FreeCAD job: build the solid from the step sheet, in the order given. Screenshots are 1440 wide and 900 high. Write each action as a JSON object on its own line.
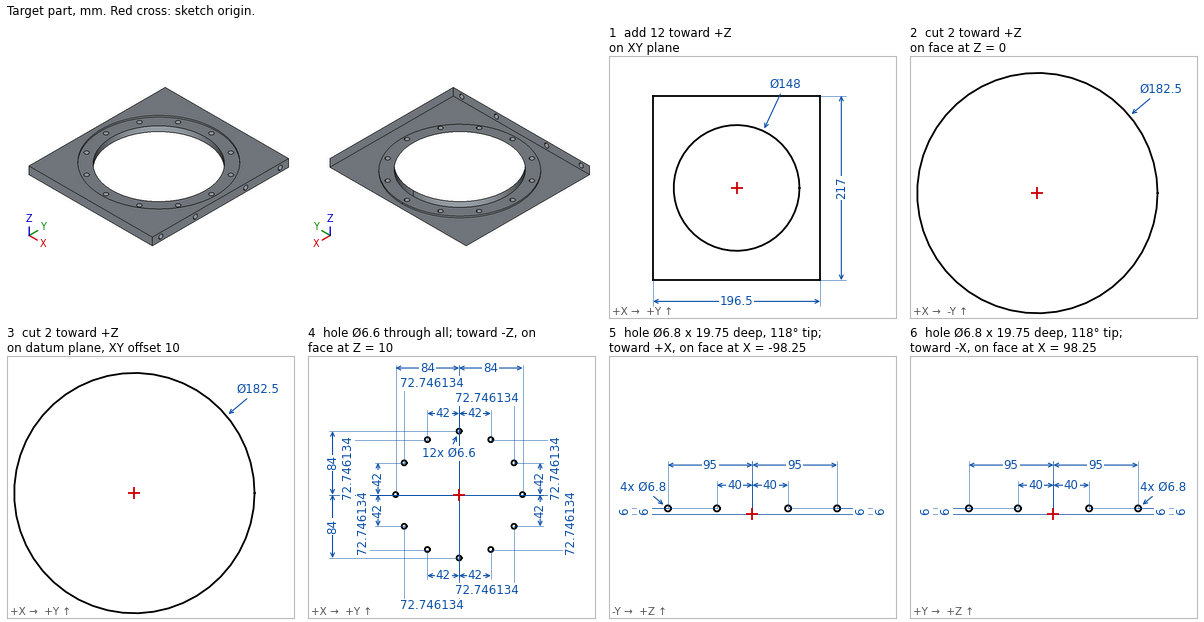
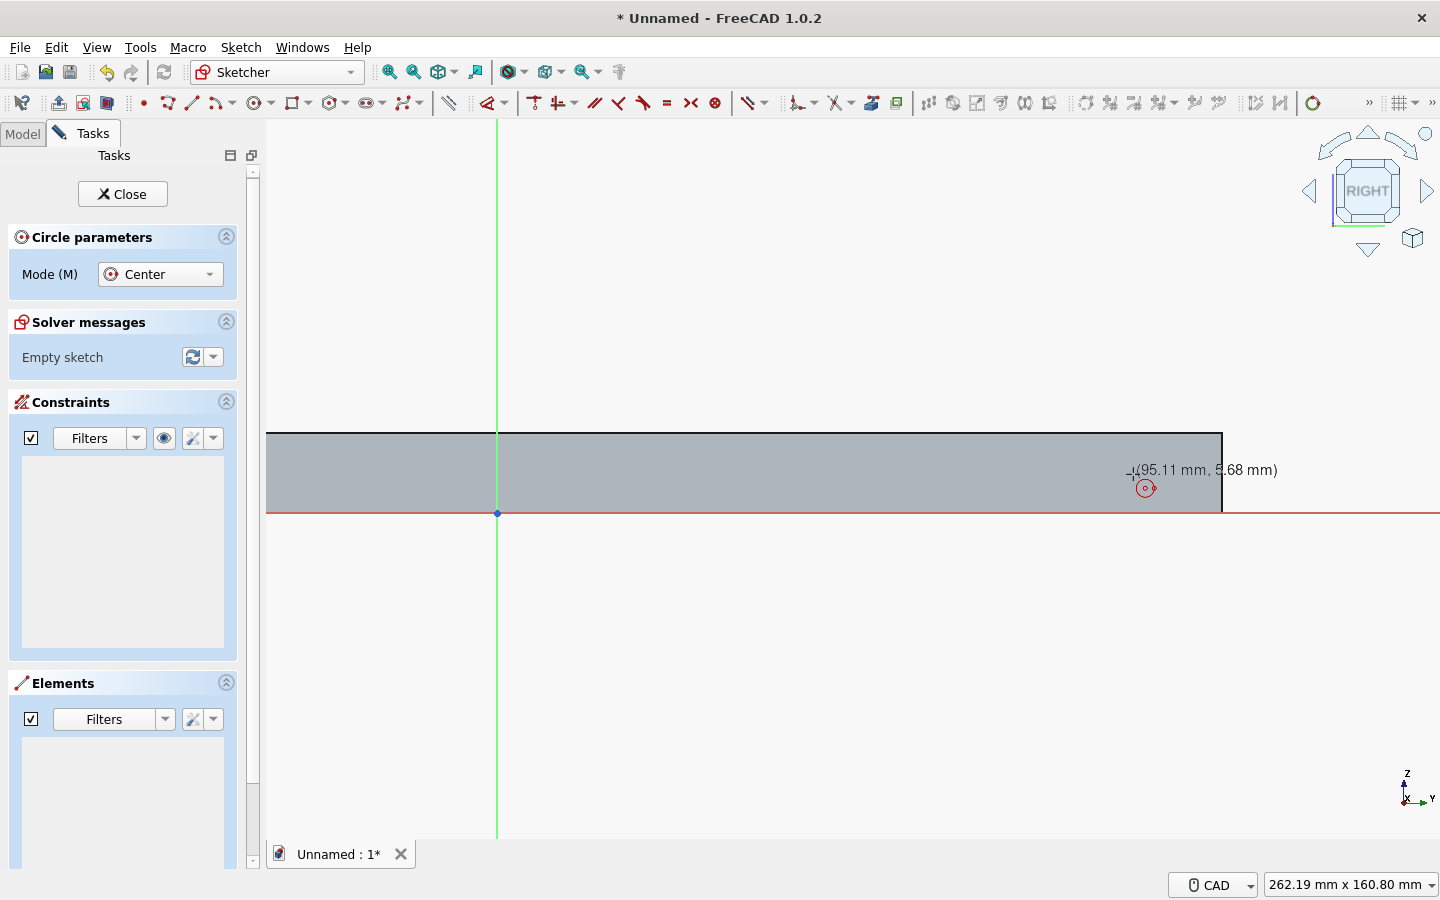
{"action": "left_click", "coordinate": [1132, 473]}
{"action": "mouse_move", "coordinate": [1148, 457]}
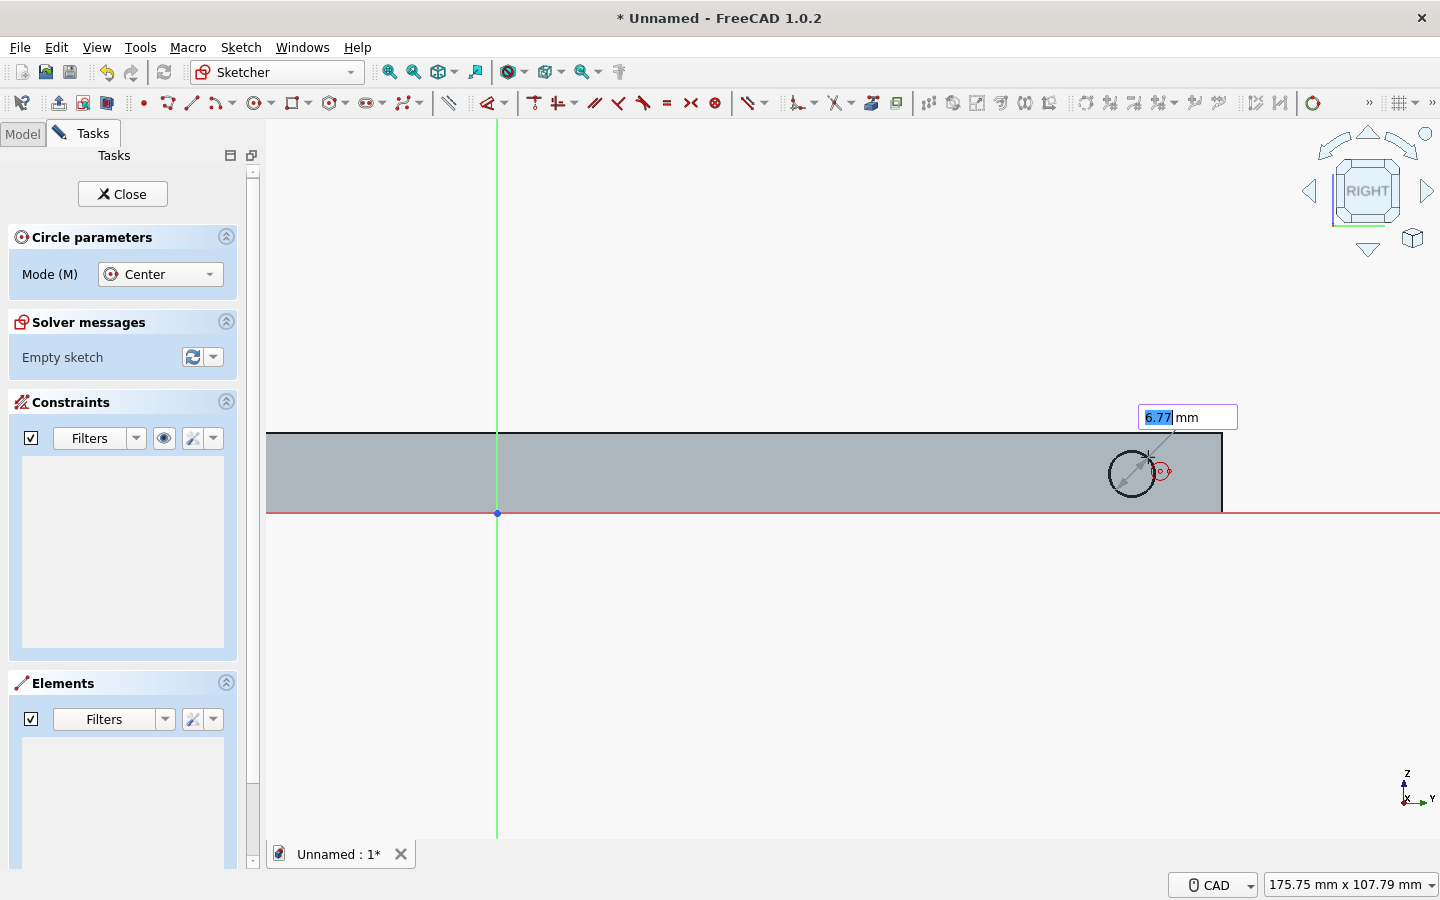
{"action": "type", "text": "6.8"}
{"action": "key", "text": "Return"}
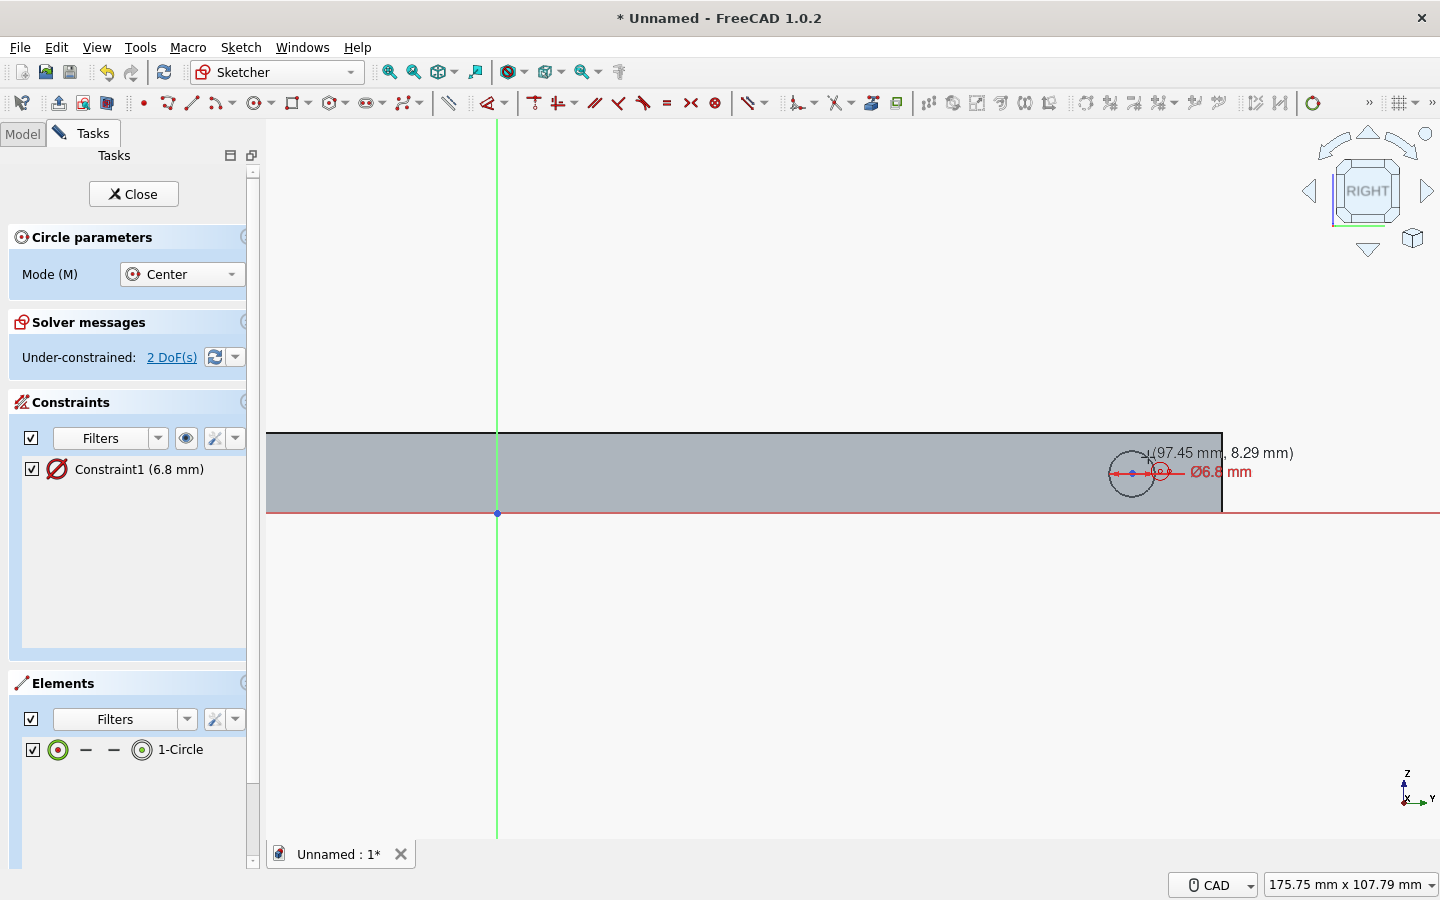
{"action": "left_click", "coordinate": [764, 473]}
{"action": "mouse_move", "coordinate": [780, 457]}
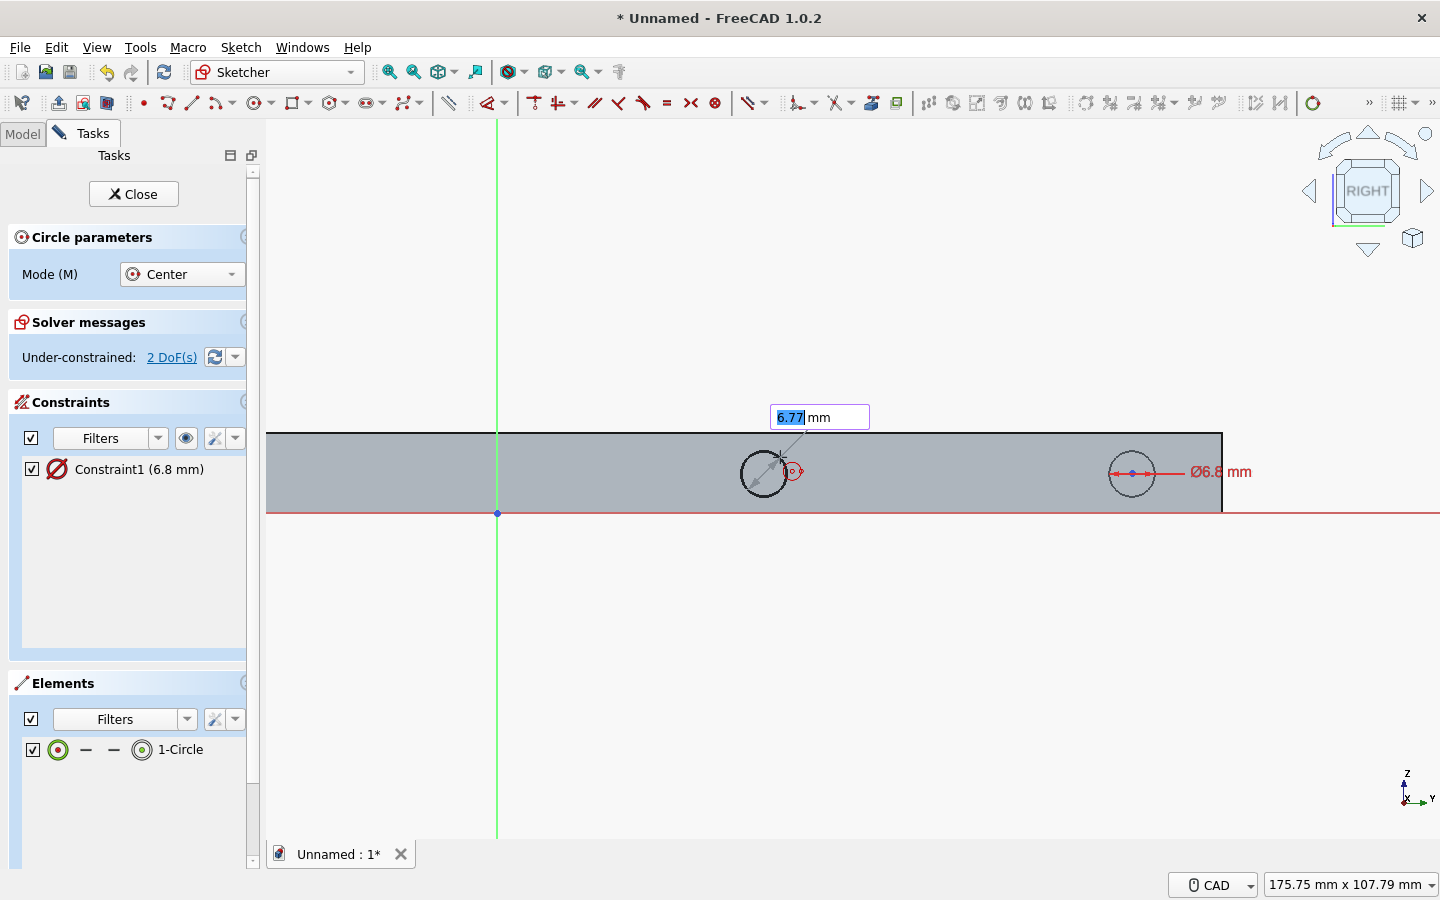
{"action": "type", "text": "6.8"}
{"action": "key", "text": "Return"}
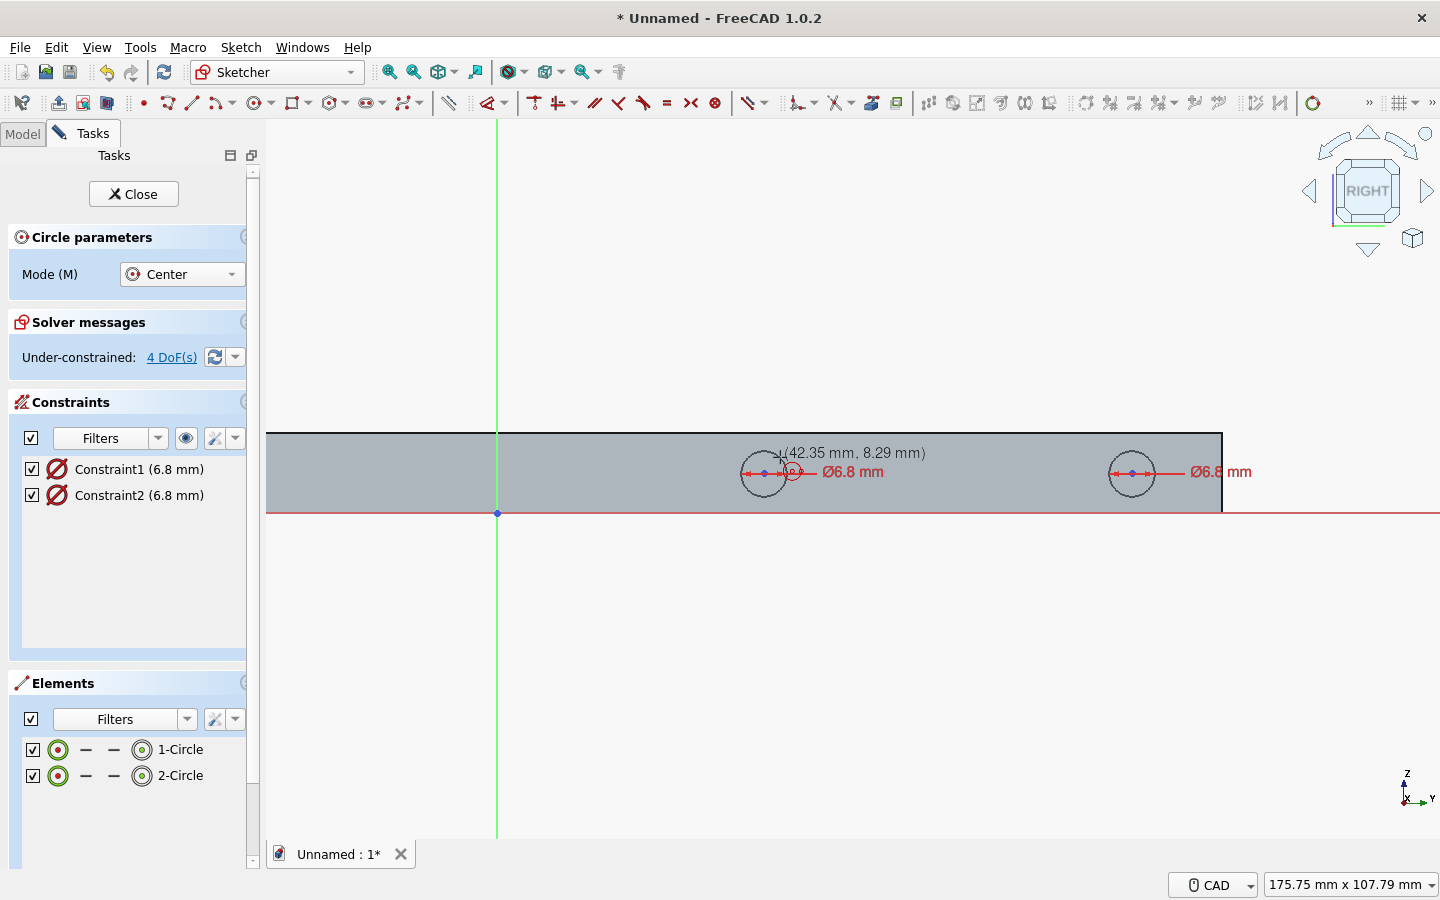
{"action": "scroll", "coordinate": [1134, 475], "scroll_direction": "down", "scroll_amount": 3}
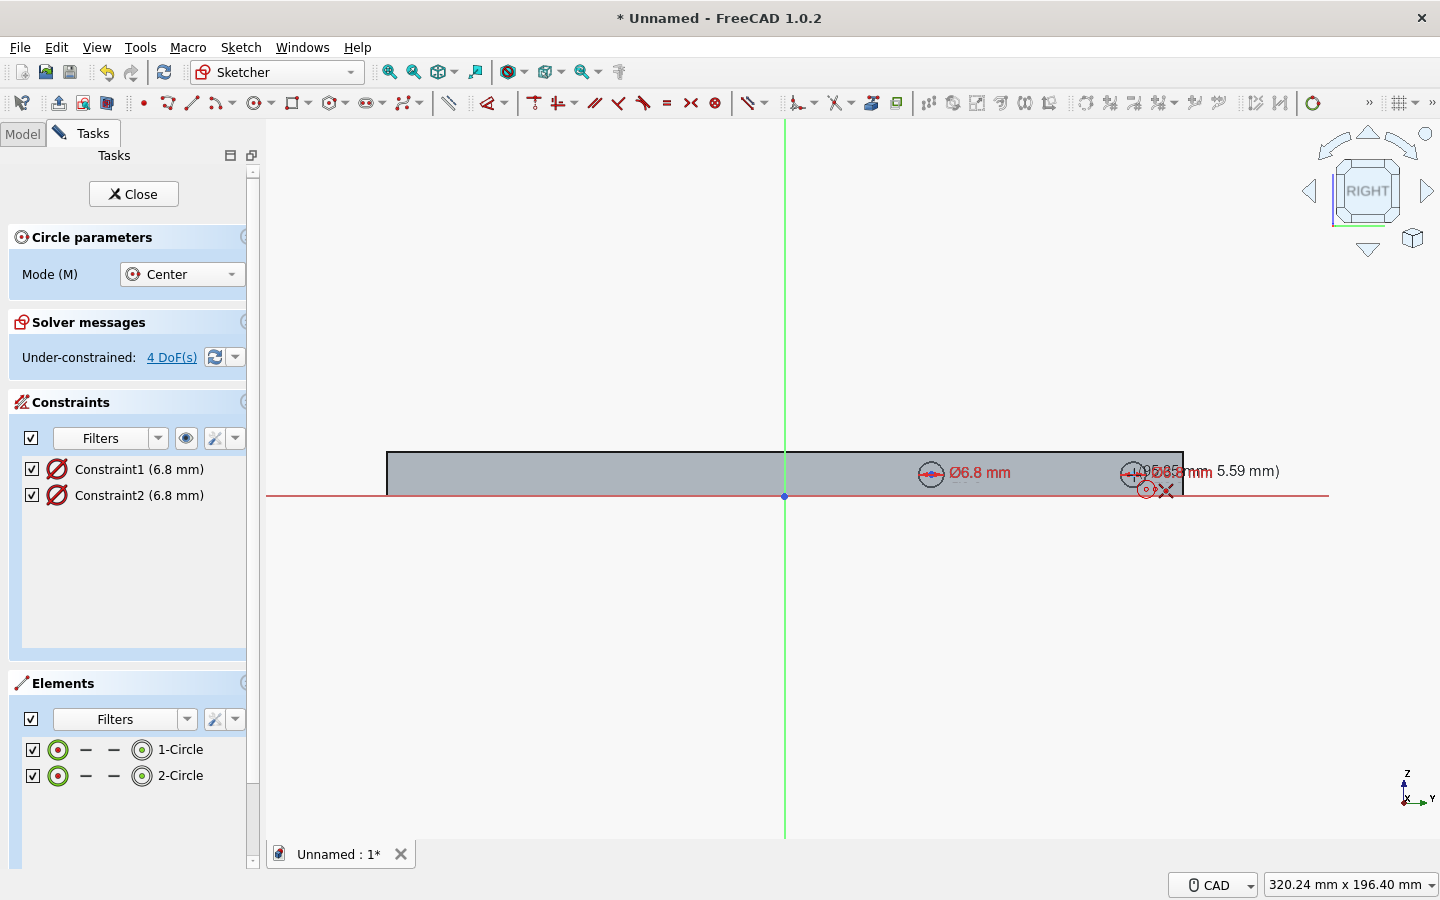
{"action": "scroll", "coordinate": [638, 474], "scroll_direction": "up", "scroll_amount": 3}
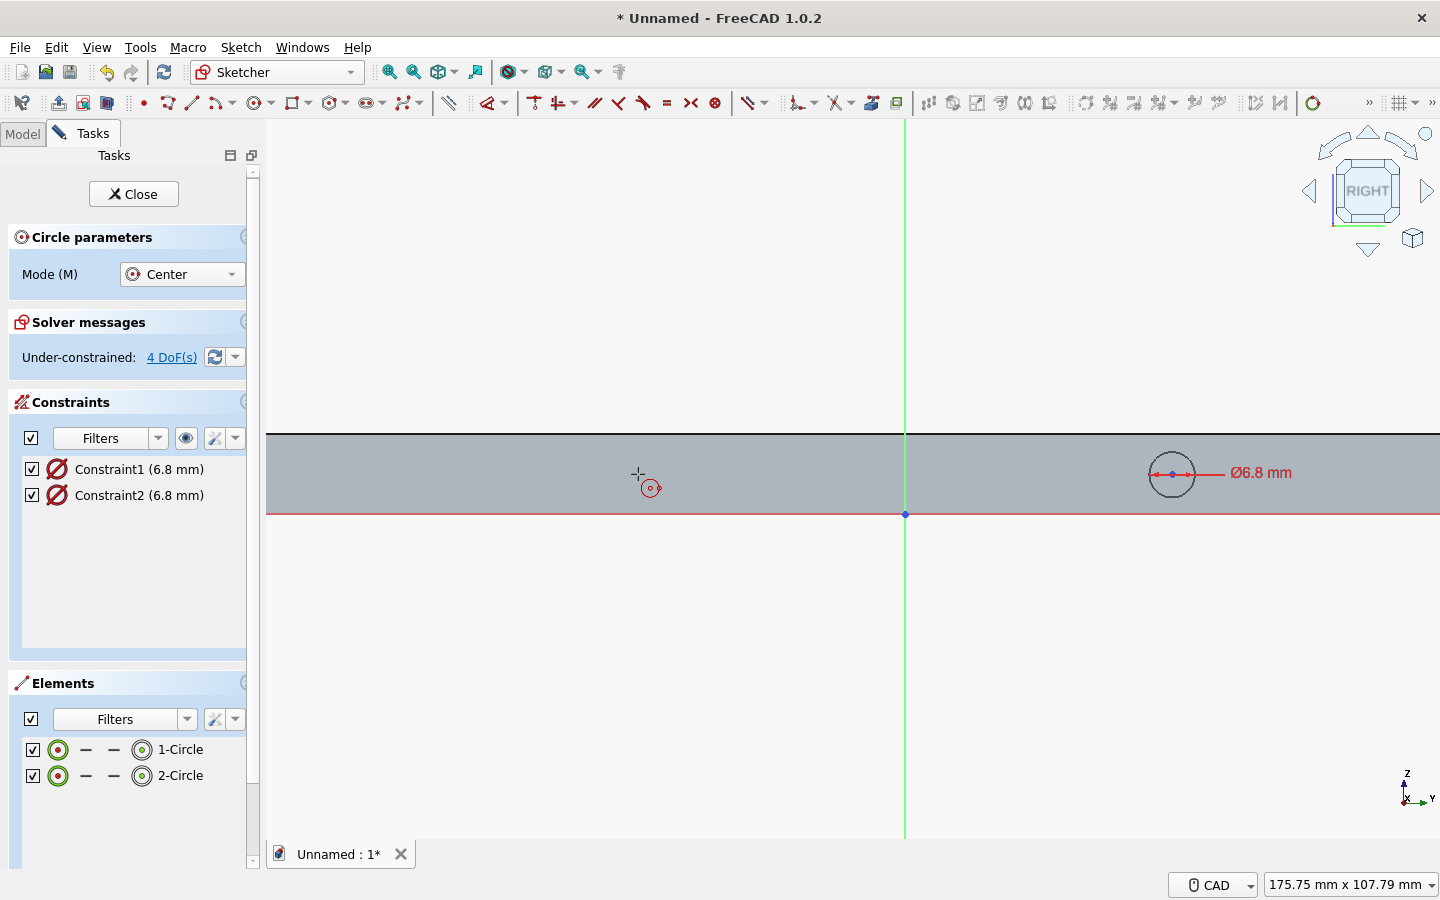
{"action": "left_click", "coordinate": [638, 474]}
{"action": "mouse_move", "coordinate": [654, 458]}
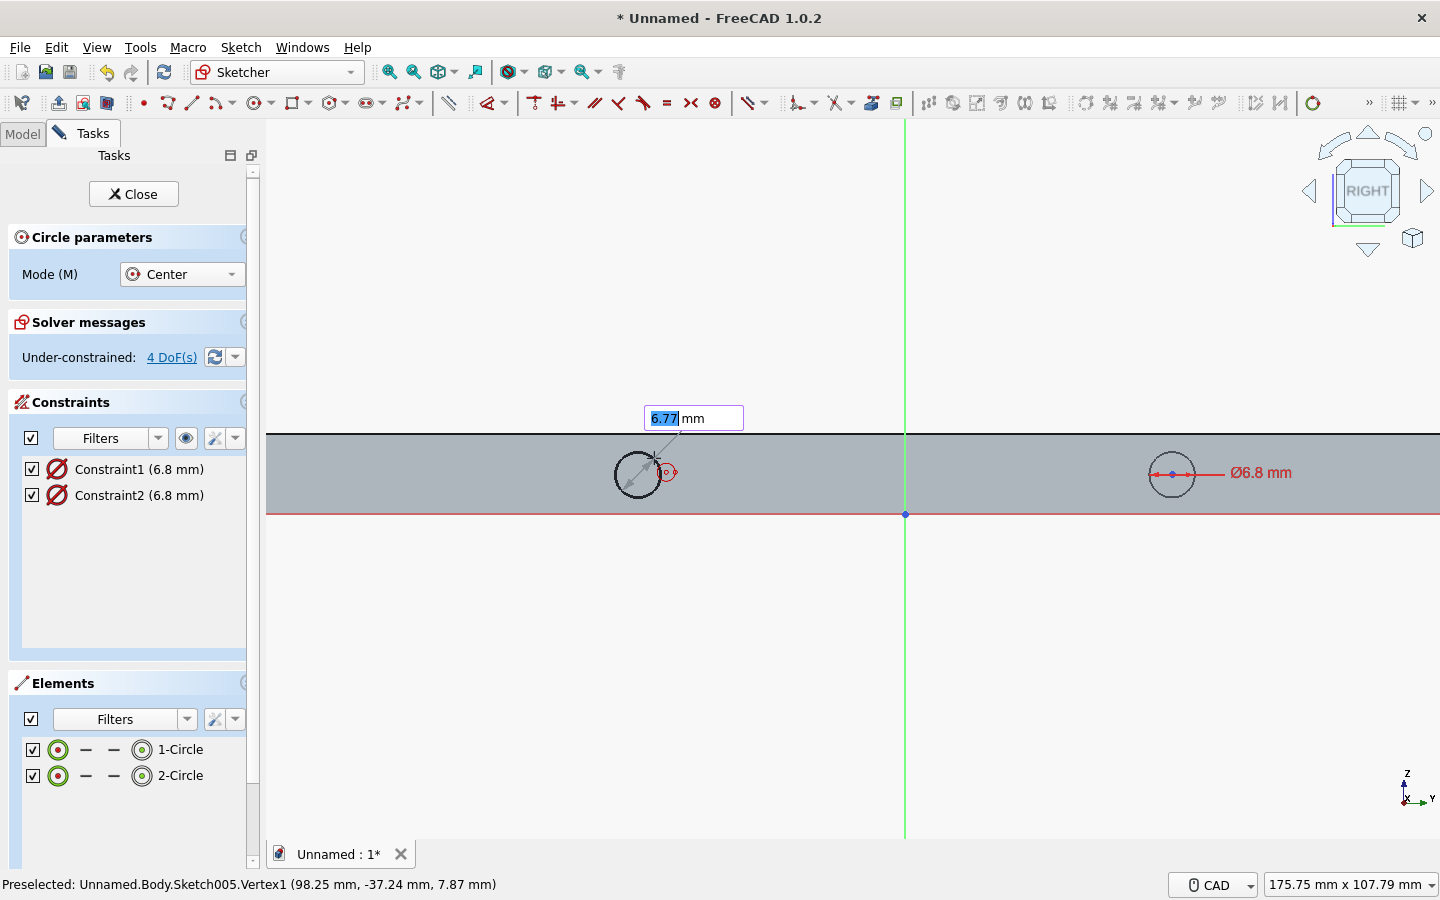
{"action": "type", "text": "6.8"}
{"action": "key", "text": "Return"}